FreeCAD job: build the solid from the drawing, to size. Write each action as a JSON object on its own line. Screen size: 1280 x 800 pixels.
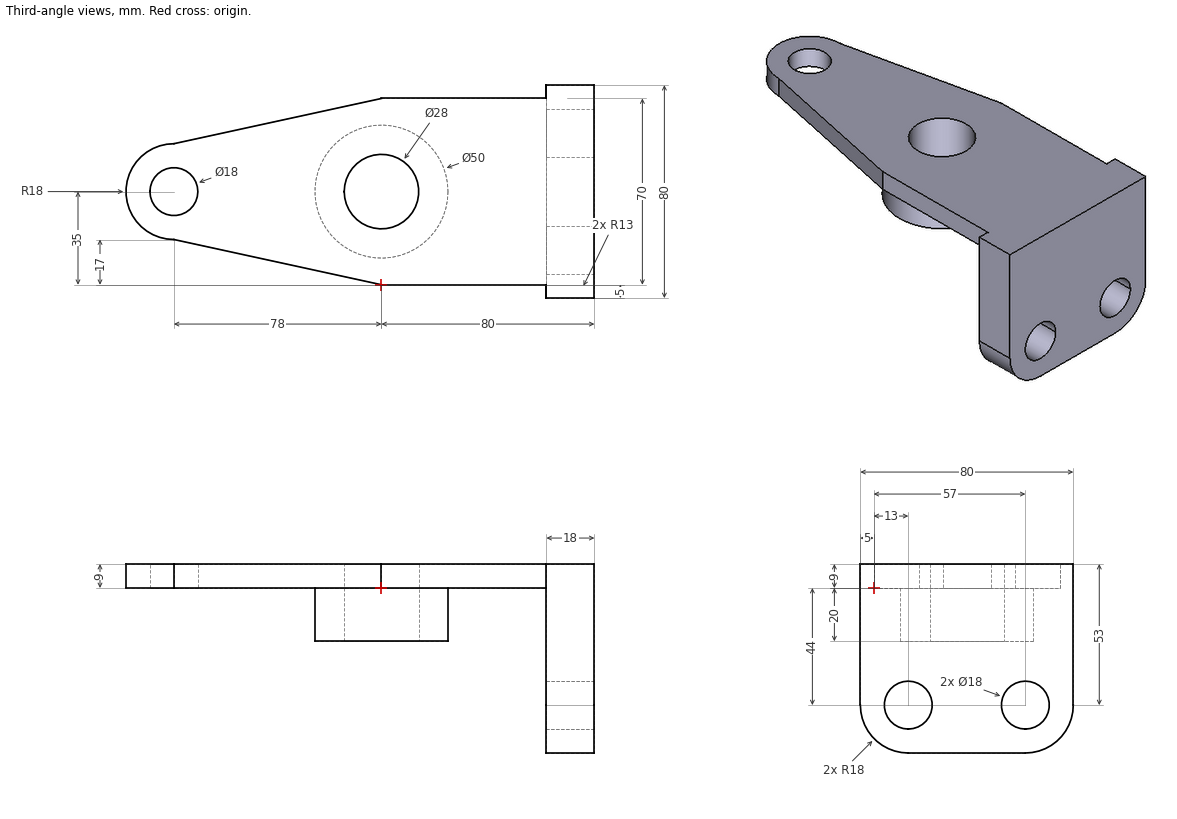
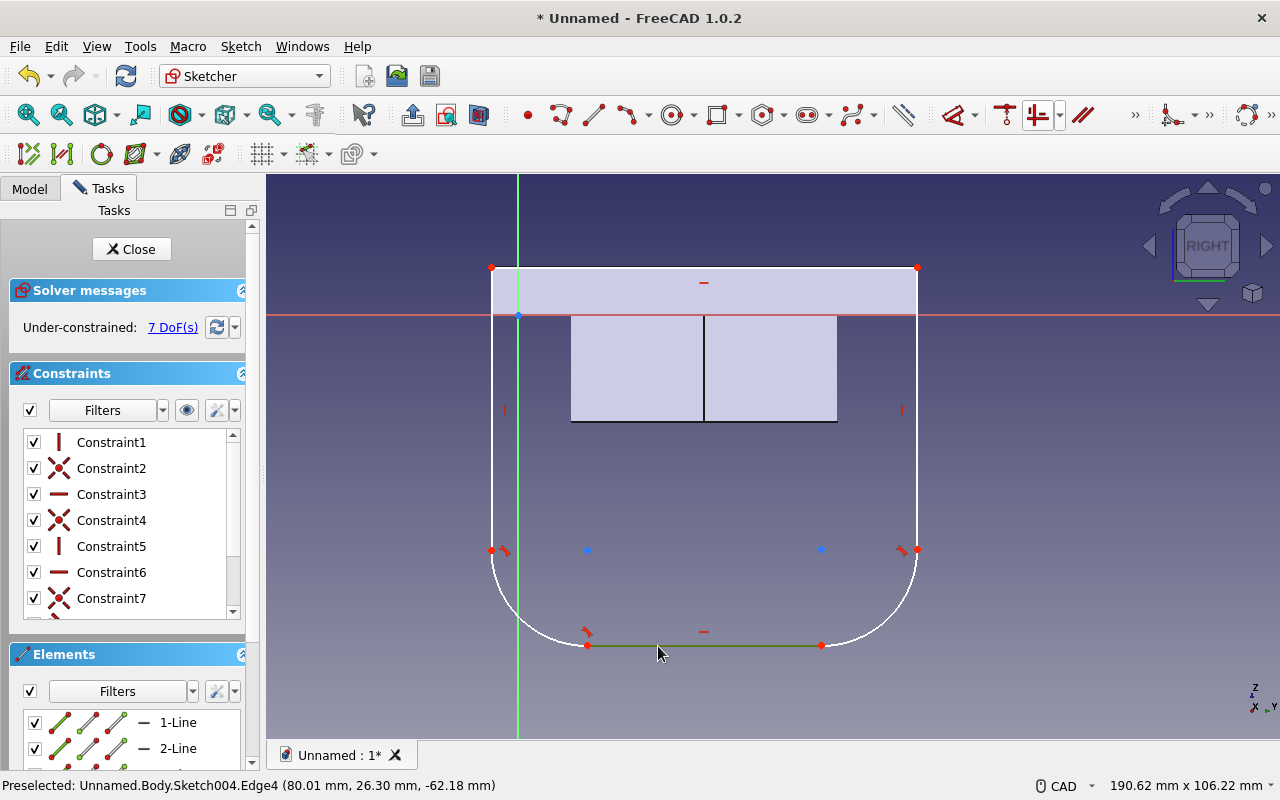
{"action": "left_click", "coordinate": [865, 636]}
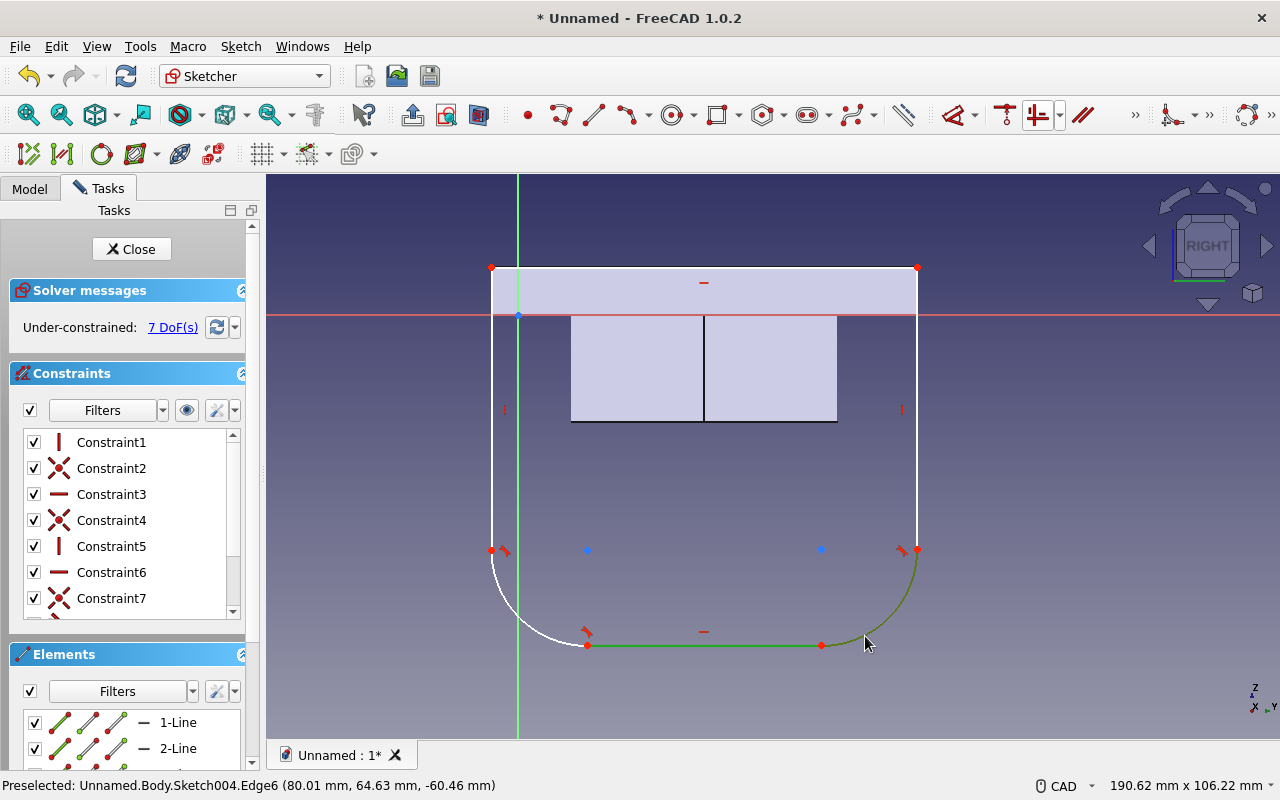
{"action": "key", "text": "t"}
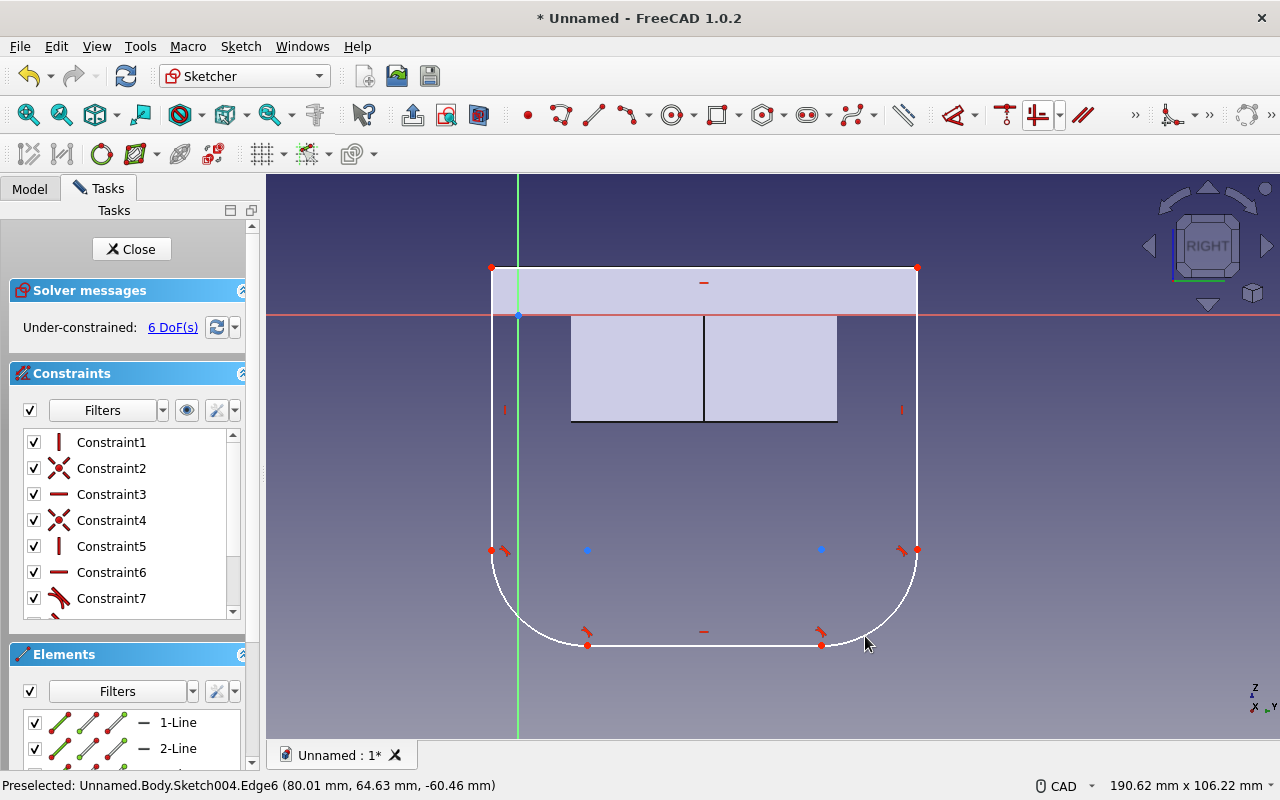
{"action": "left_click", "coordinate": [502, 594]}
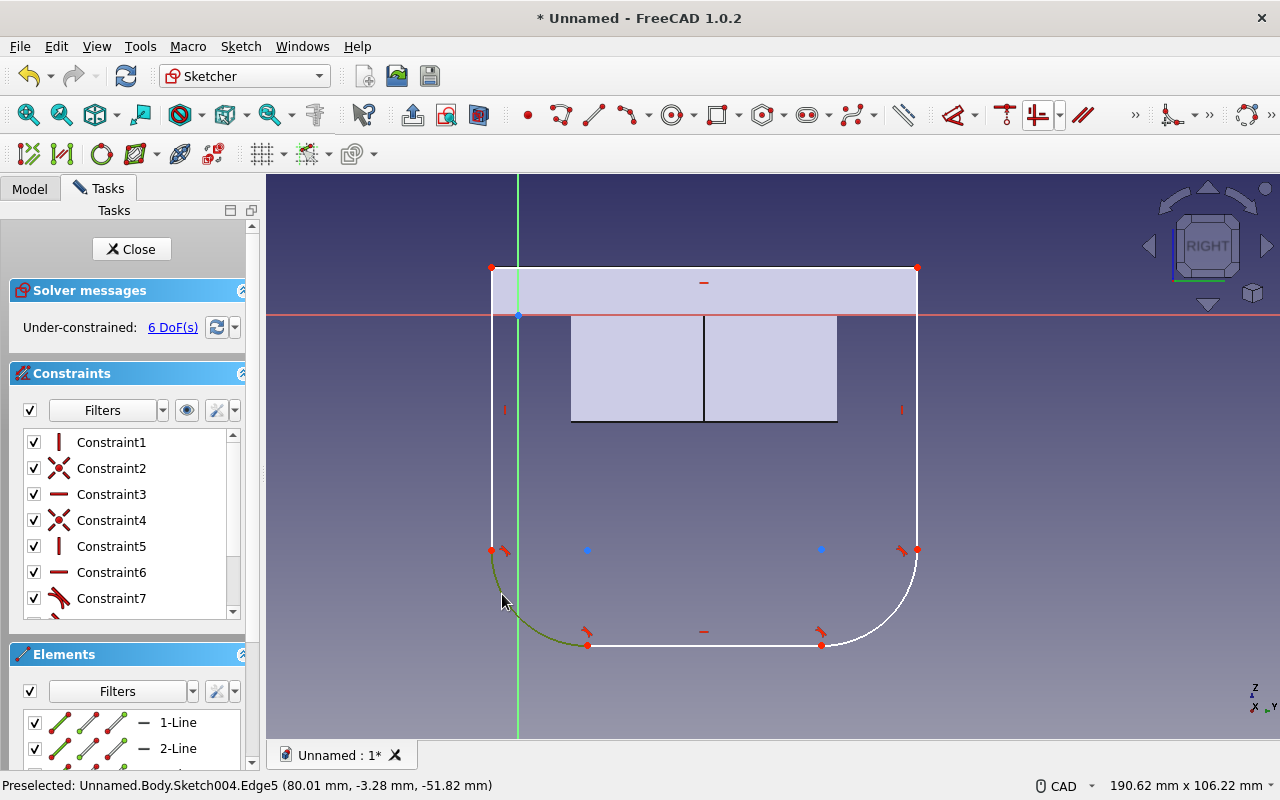
{"action": "left_click", "coordinate": [865, 636]}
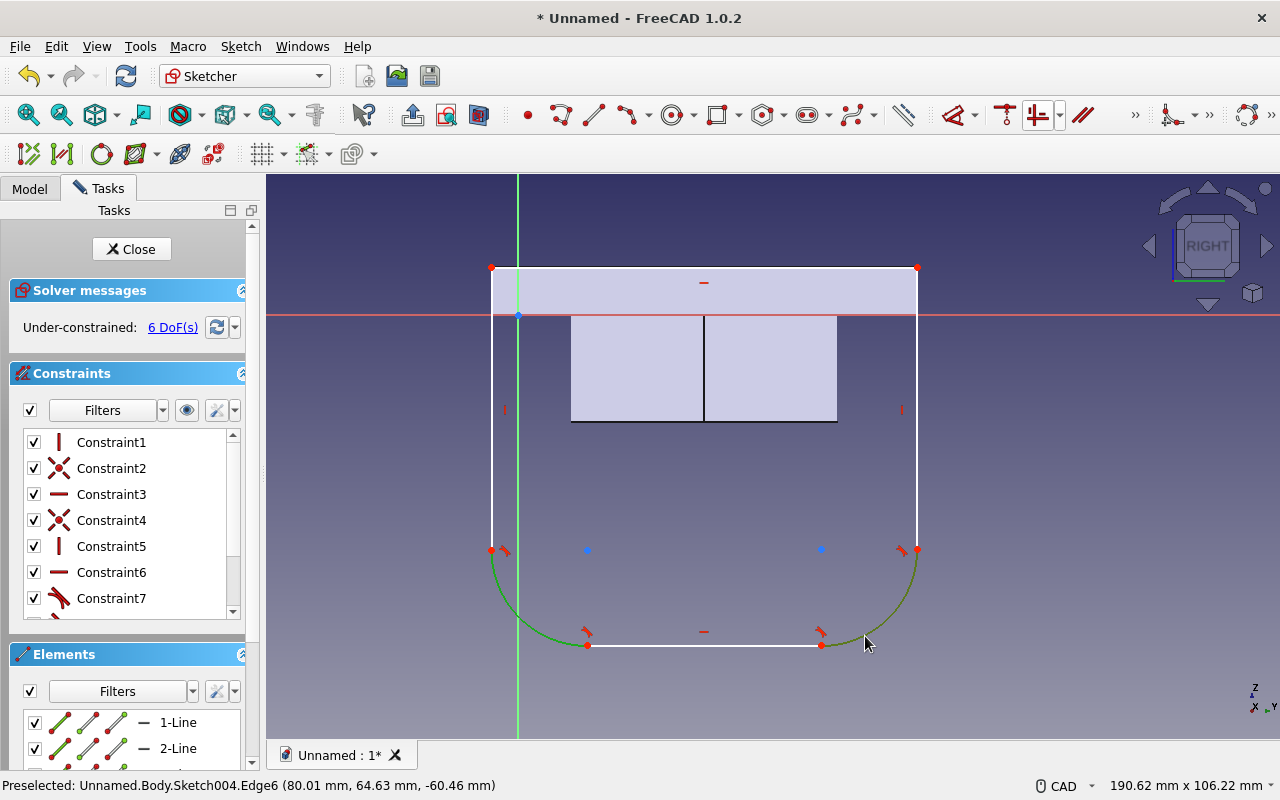
{"action": "key", "text": "e"}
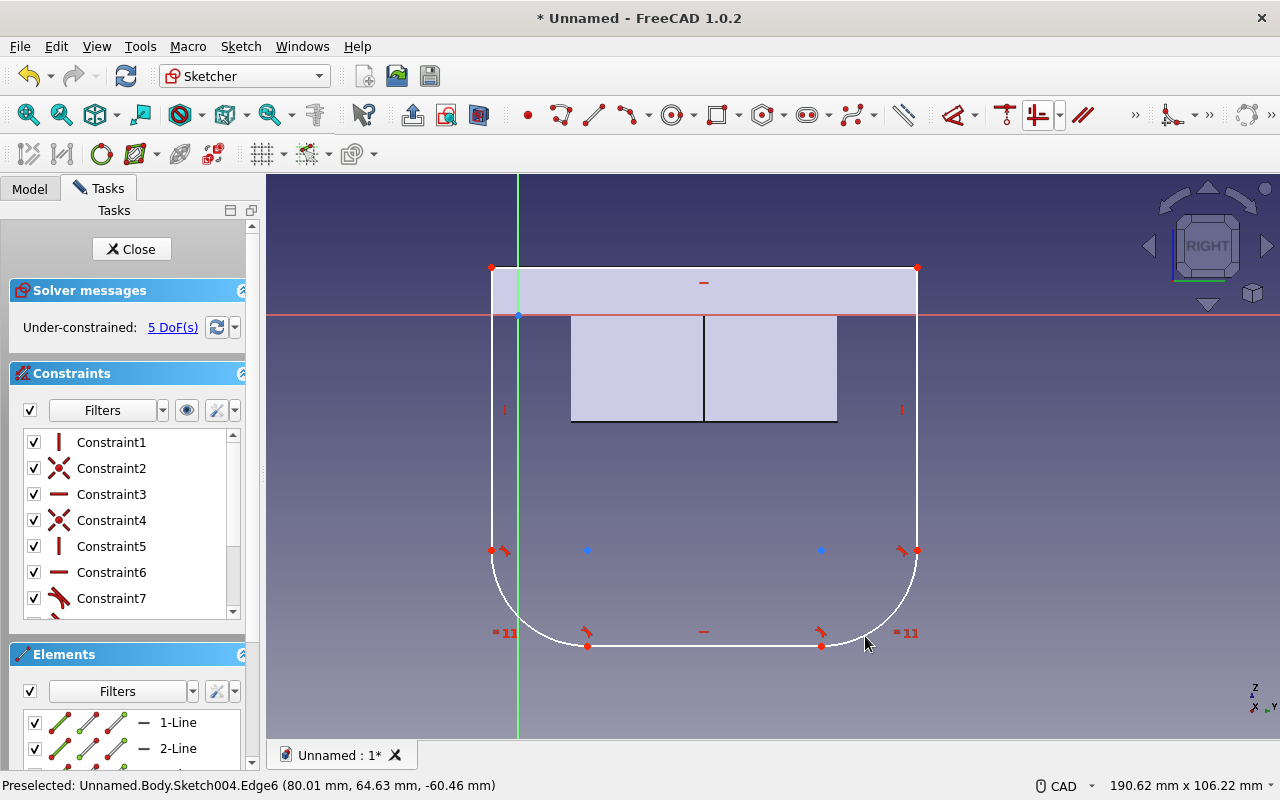
{"action": "left_click", "coordinate": [952, 116]}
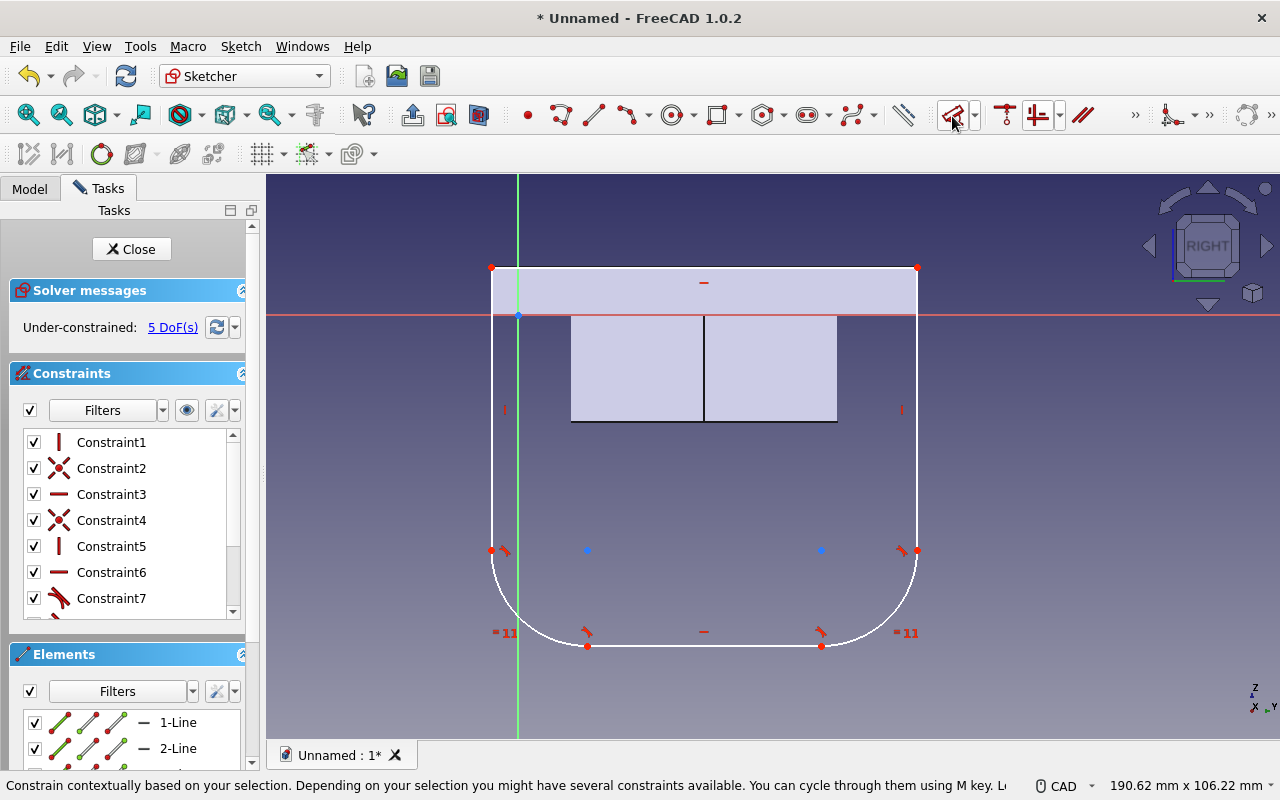
{"action": "left_click", "coordinate": [502, 594]}
{"action": "left_click", "coordinate": [474, 609]}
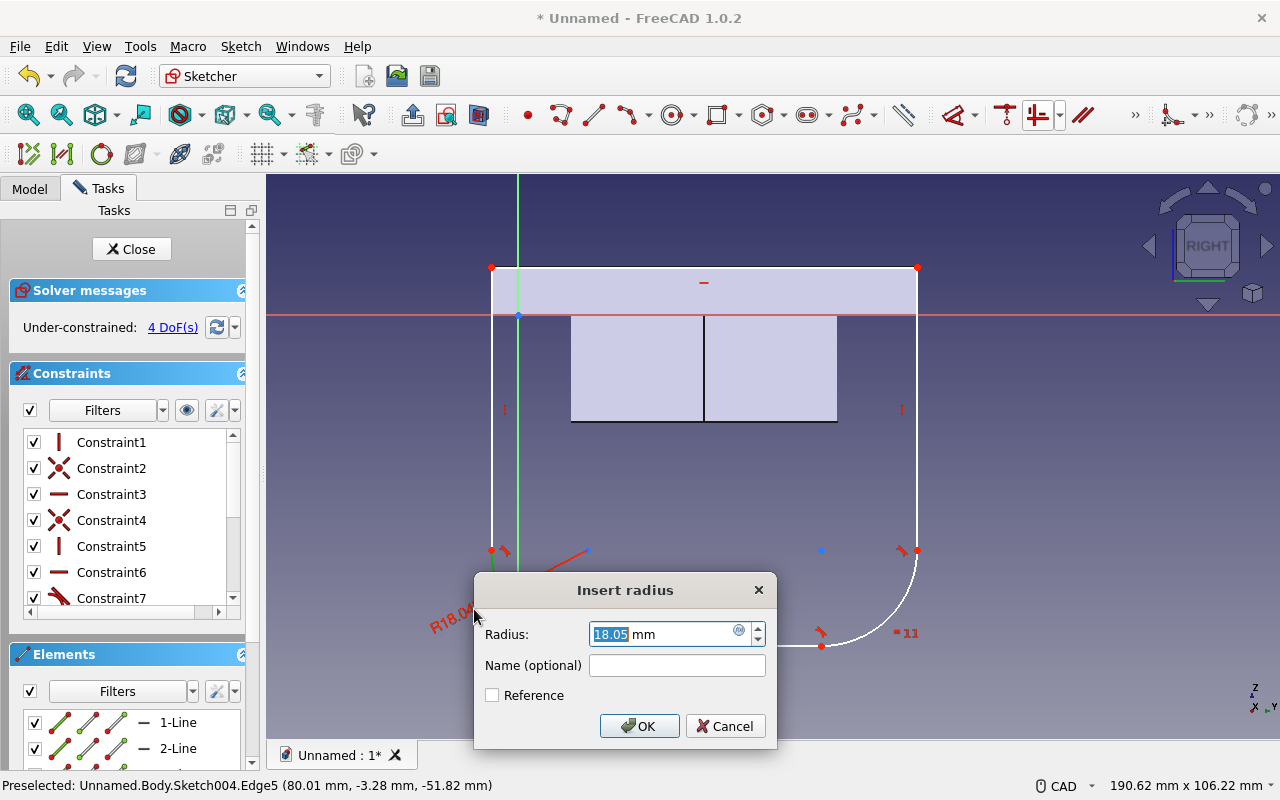
{"action": "type", "text": "18"}
{"action": "key", "text": "Return"}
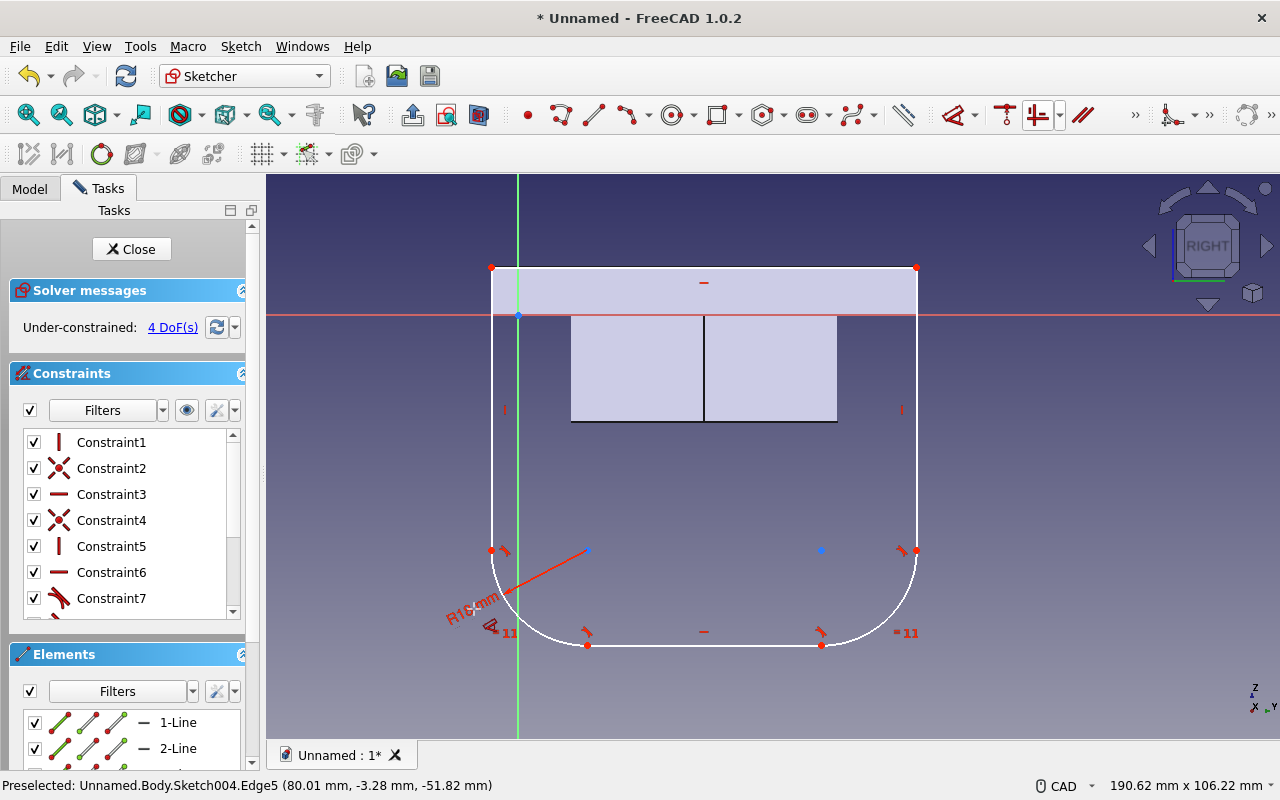
{"action": "left_click", "coordinate": [917, 465]}
{"action": "left_click", "coordinate": [951, 409]}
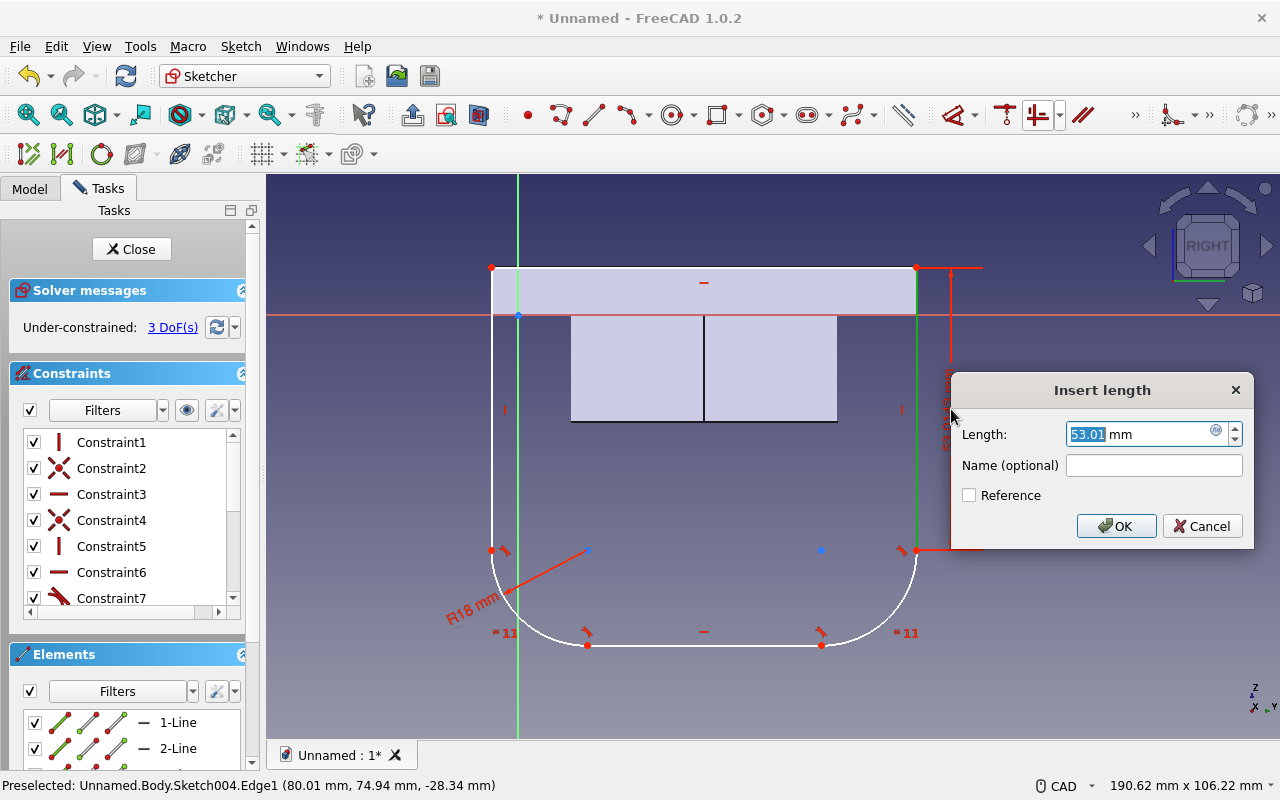
{"action": "type", "text": "53"}
{"action": "key", "text": "Return"}